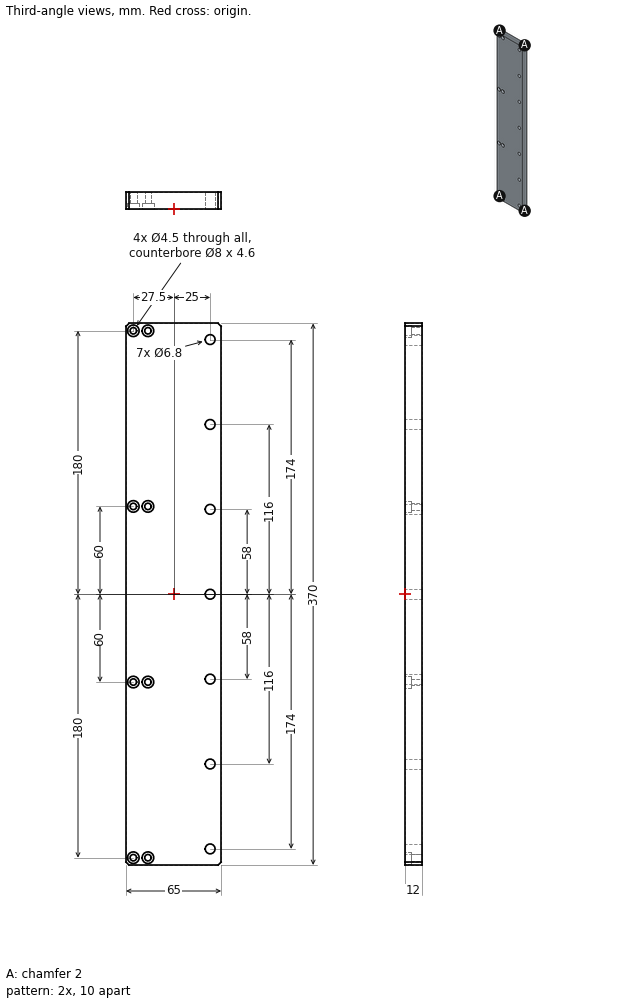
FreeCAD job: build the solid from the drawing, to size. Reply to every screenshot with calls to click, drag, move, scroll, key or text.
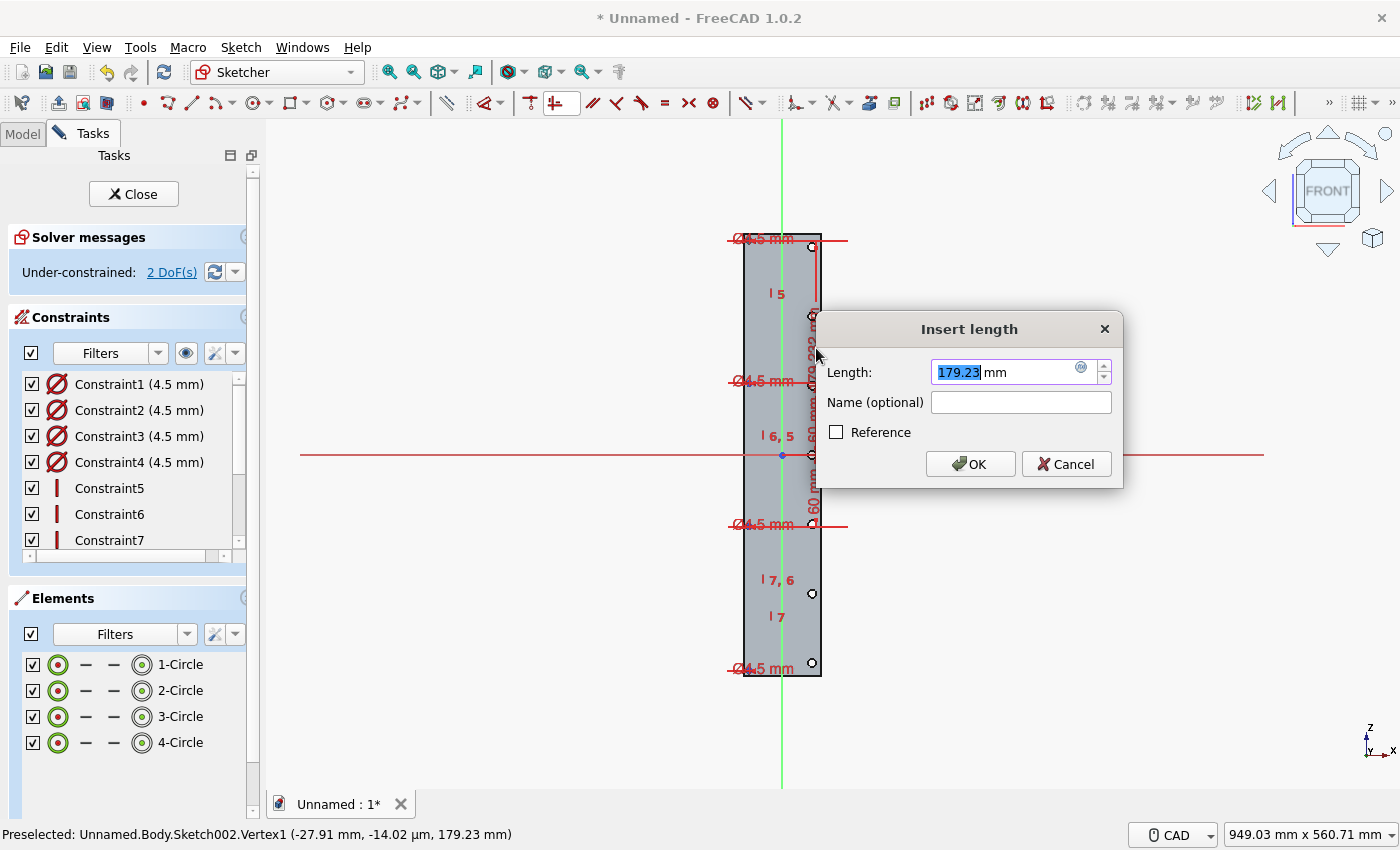
text(180)
key(Return)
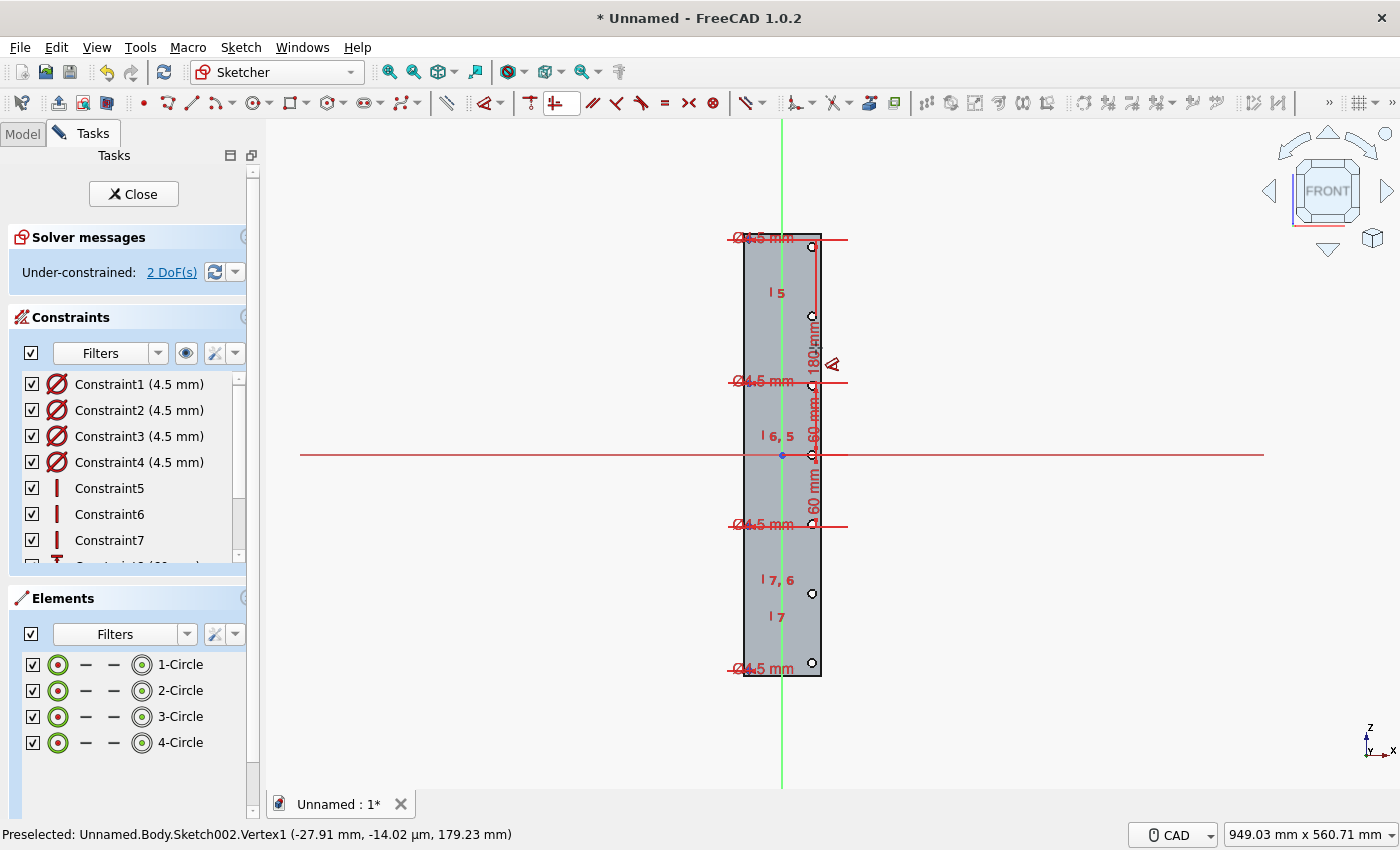
click(749, 671)
click(816, 563)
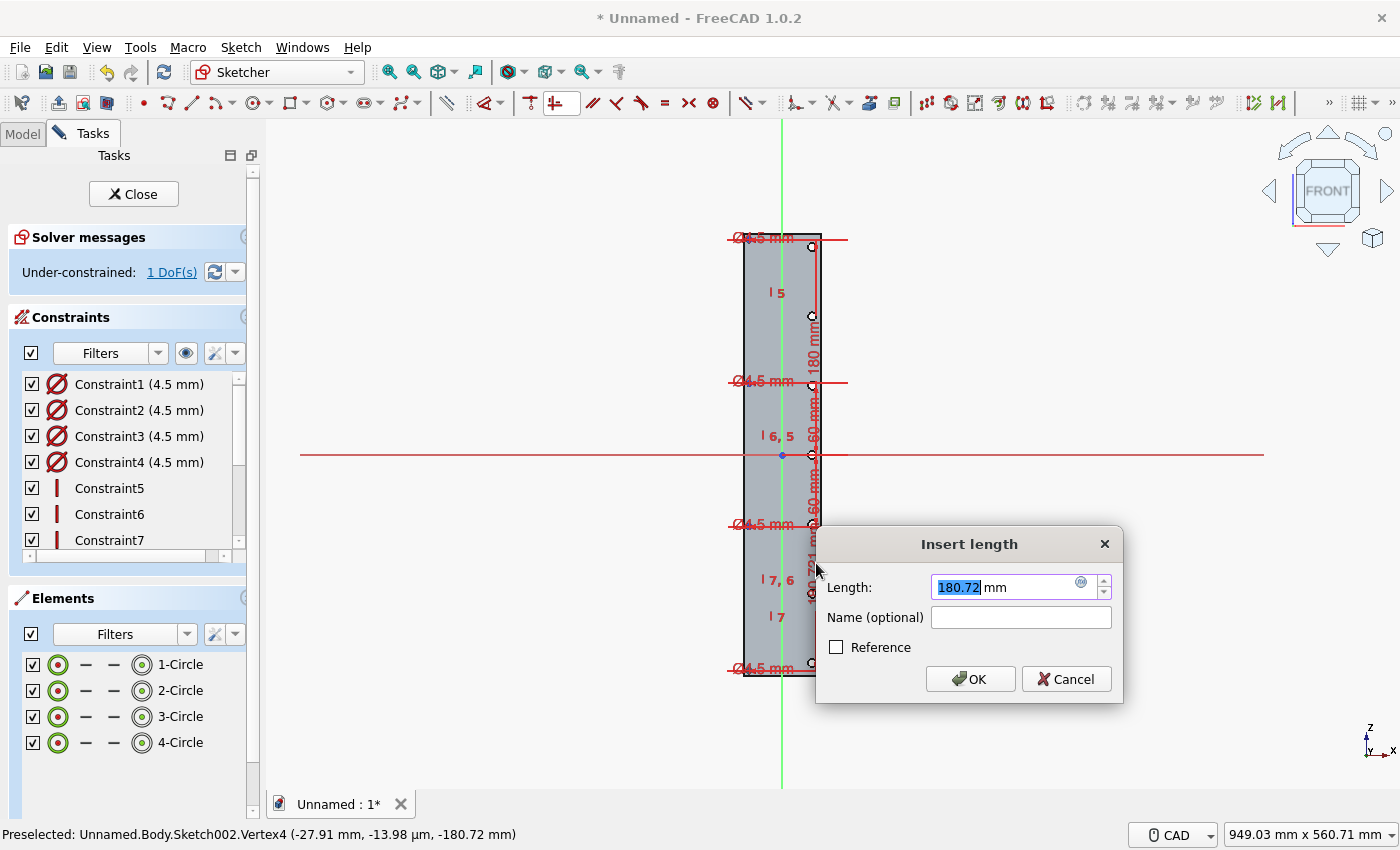
text(180)
key(Return)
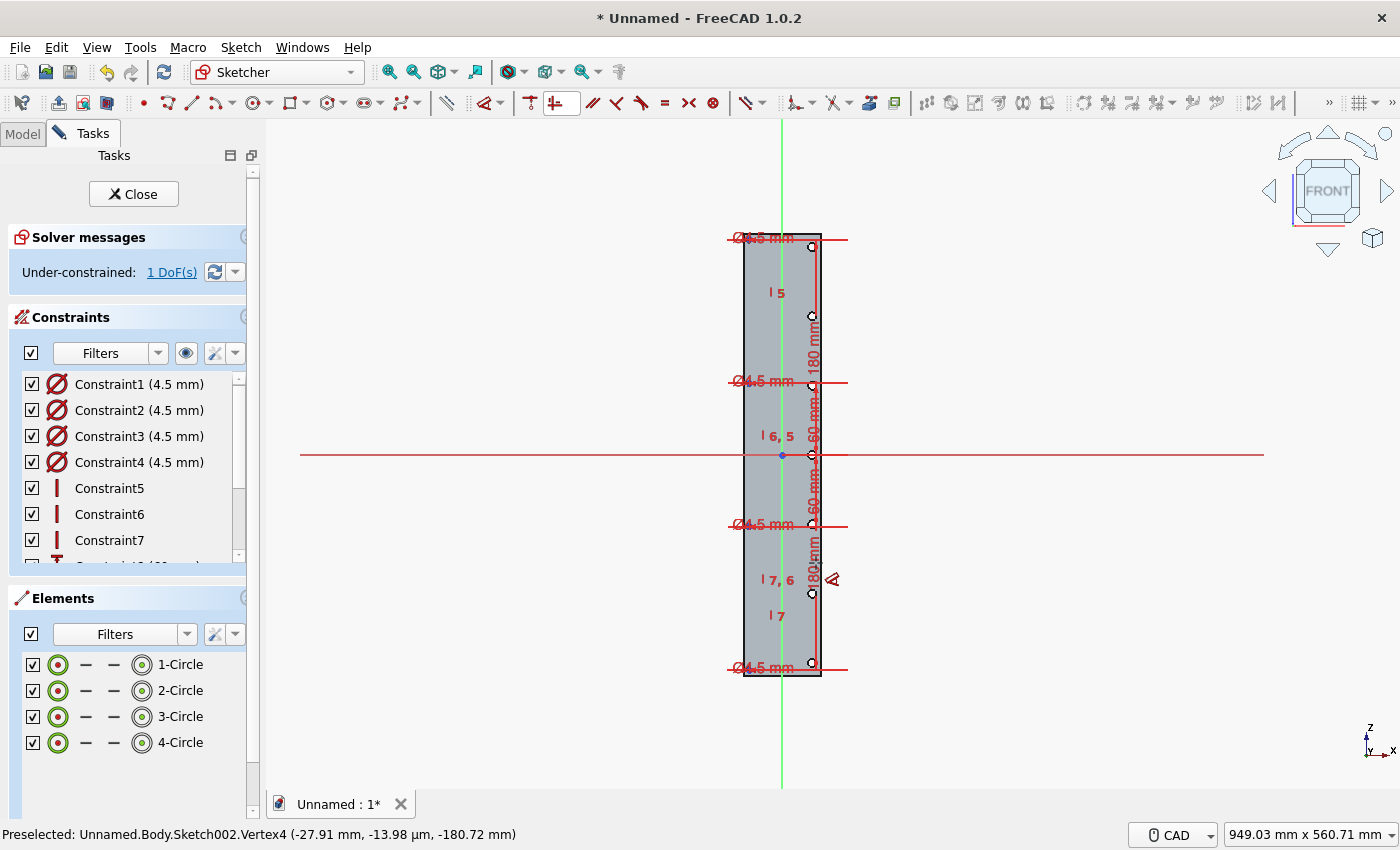
click(749, 240)
click(766, 206)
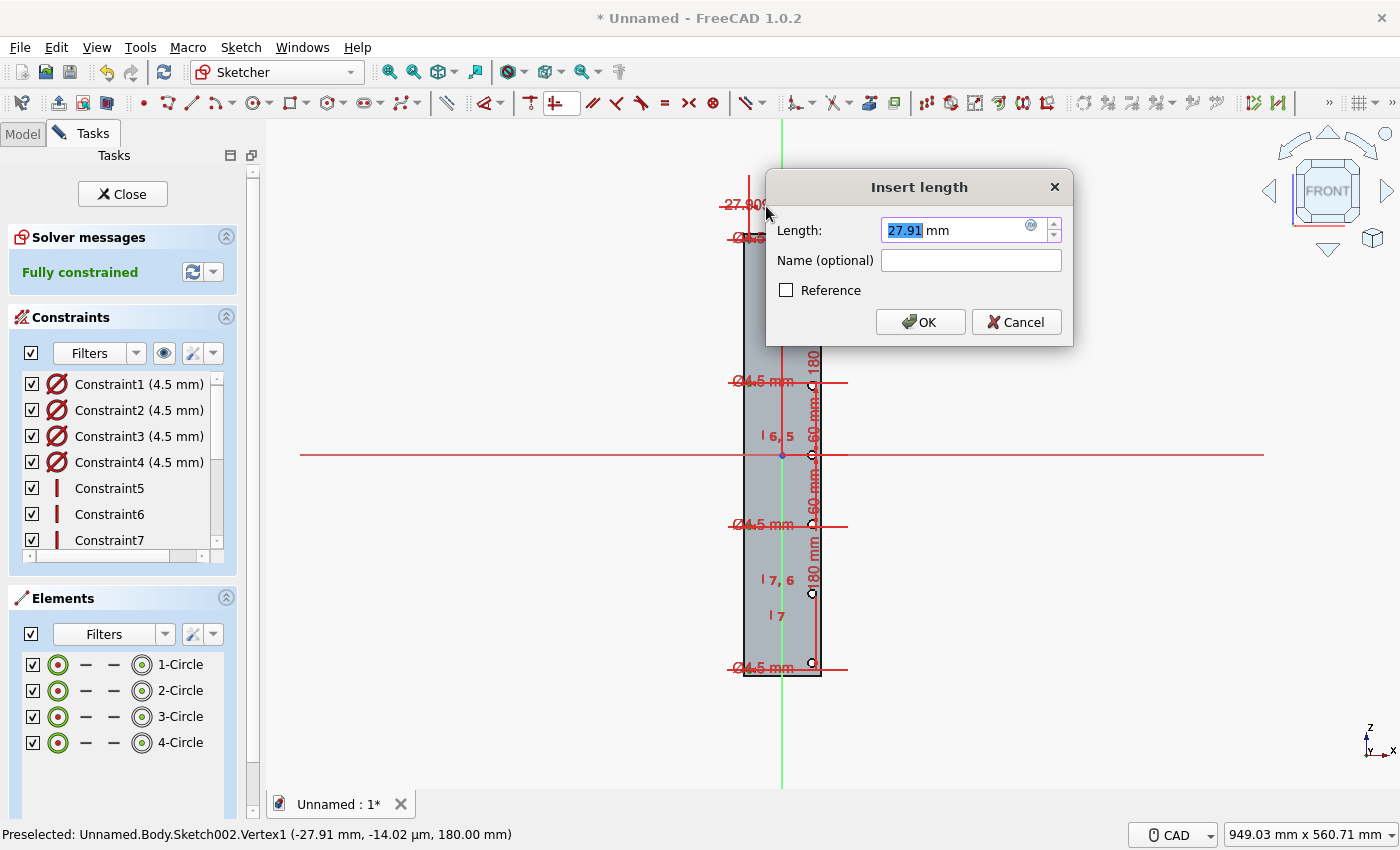
text(27.5)
key(Return)
key(Escape)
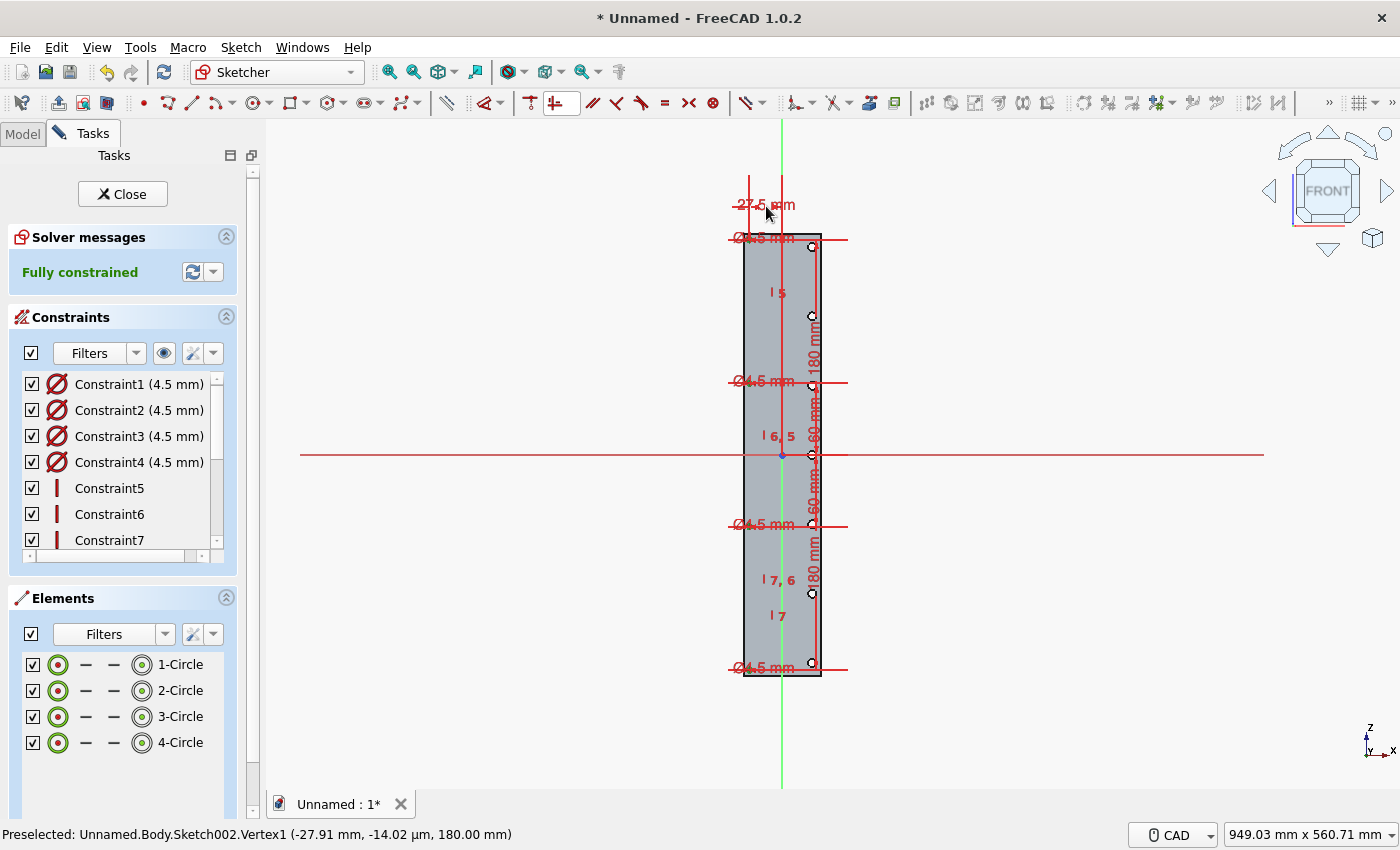
click(123, 194)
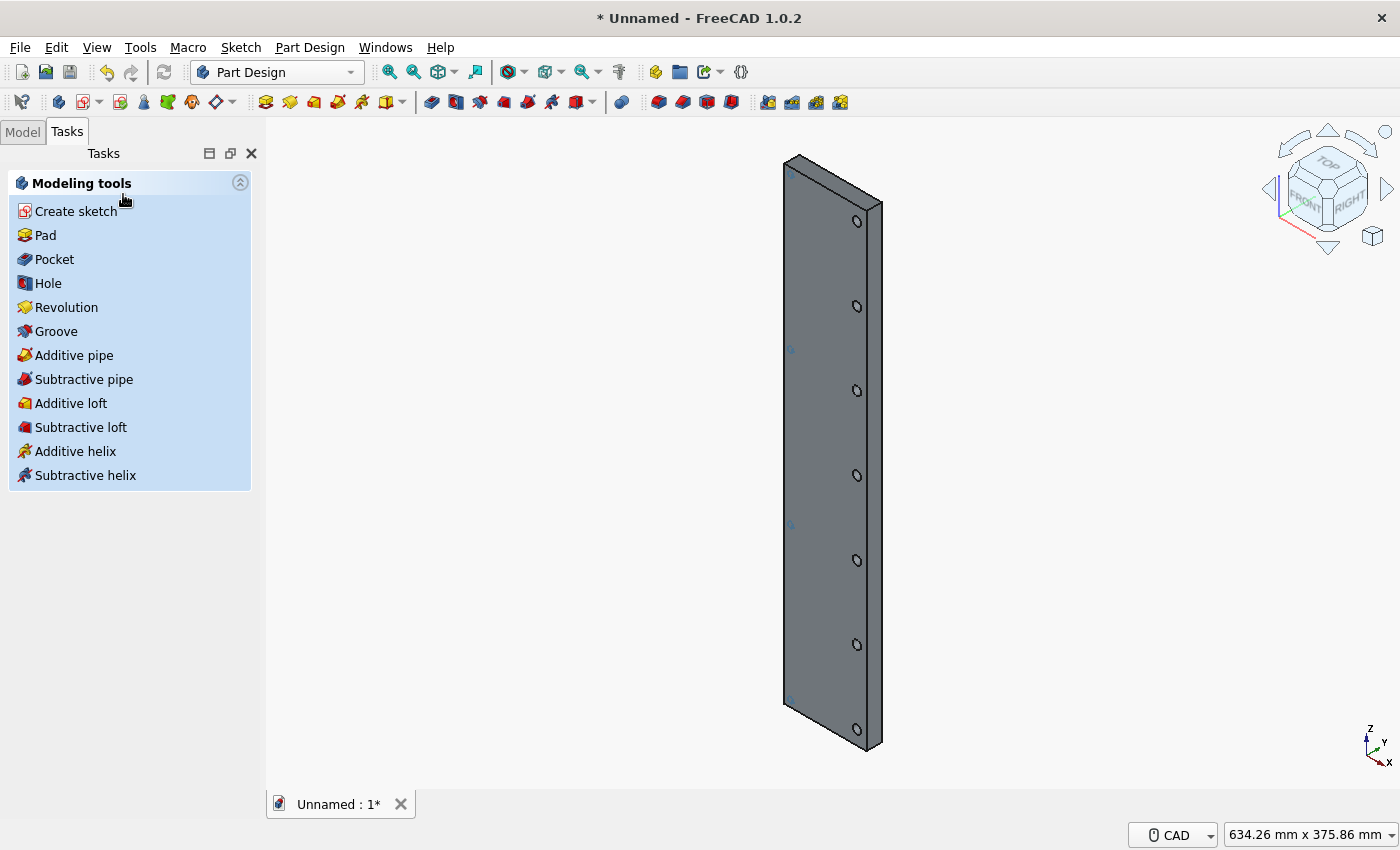
click(456, 102)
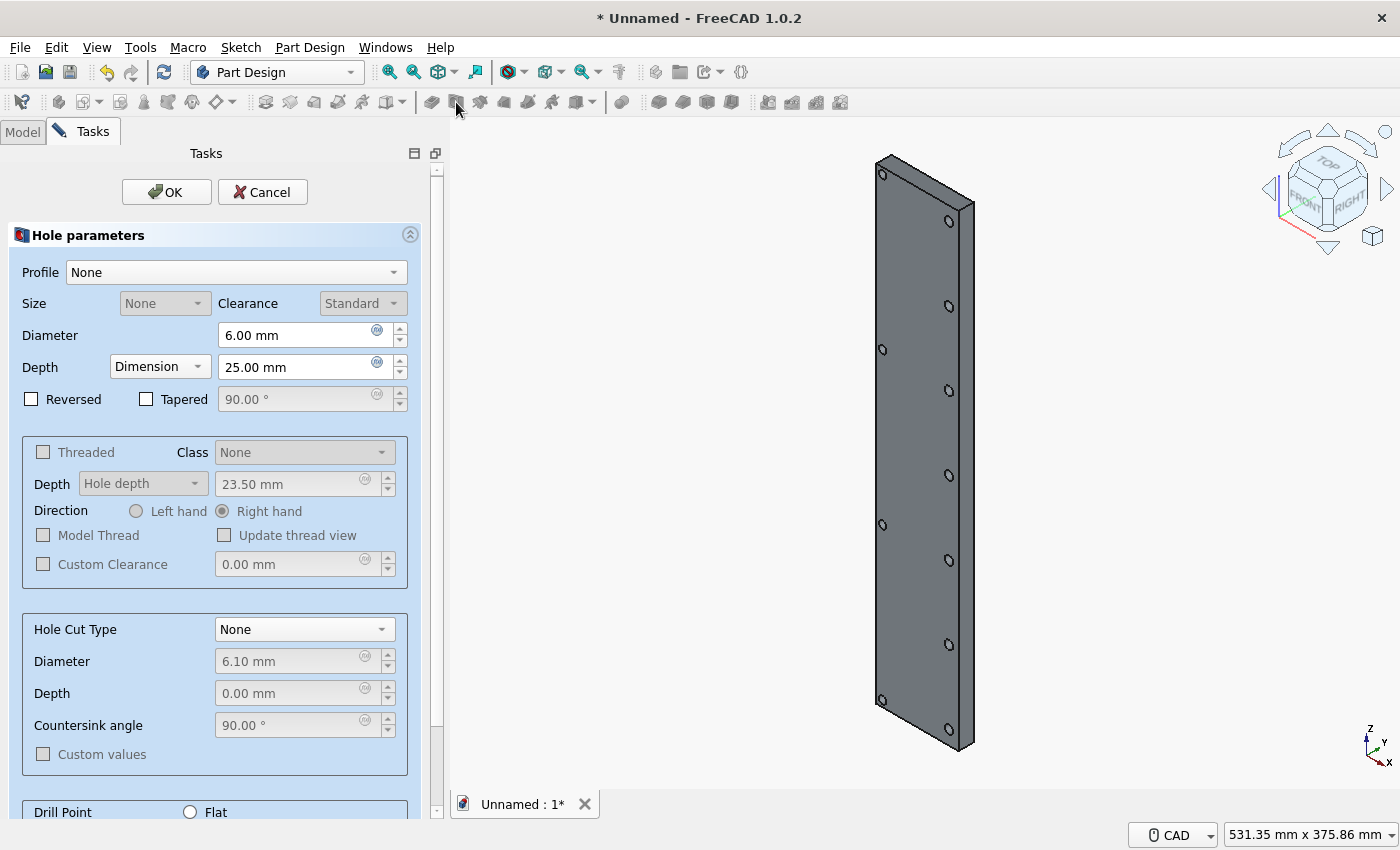
triple_click(305, 335)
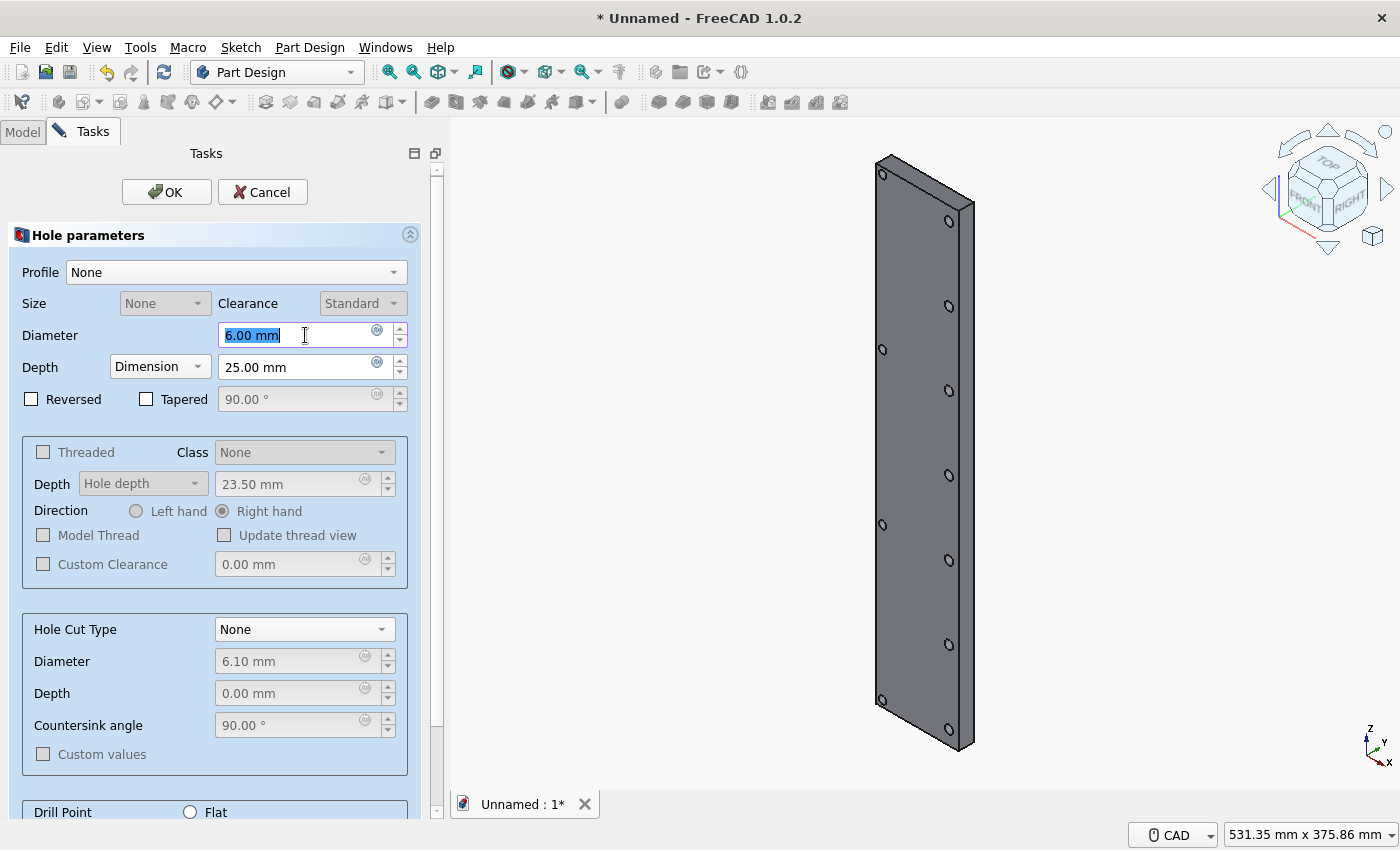
text(4.5)
key(Tab)